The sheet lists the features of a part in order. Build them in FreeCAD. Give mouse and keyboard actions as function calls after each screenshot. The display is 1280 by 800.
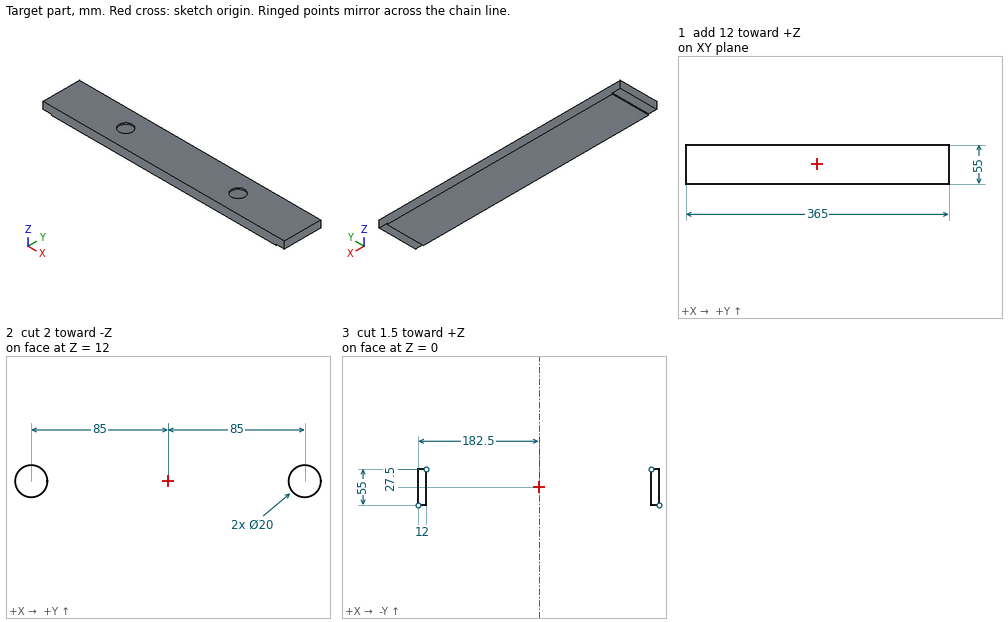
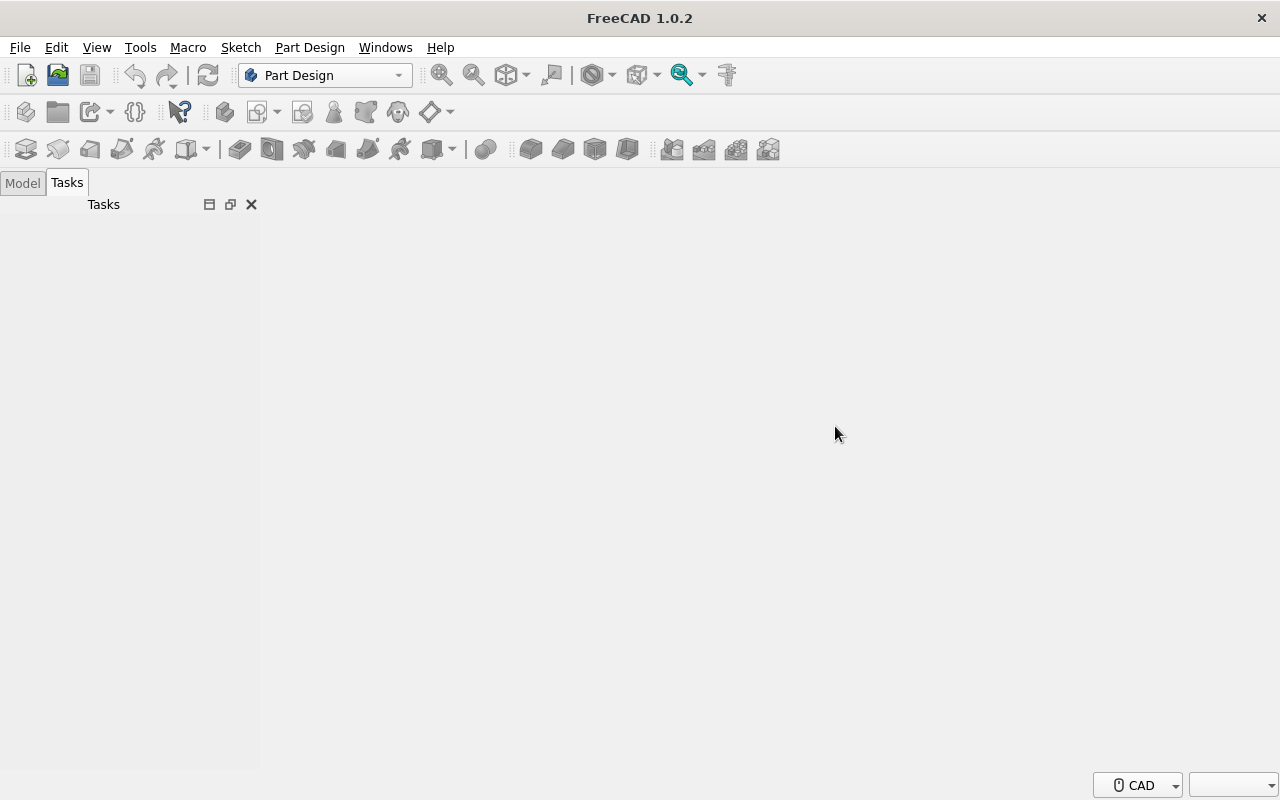
key(ctrl+n)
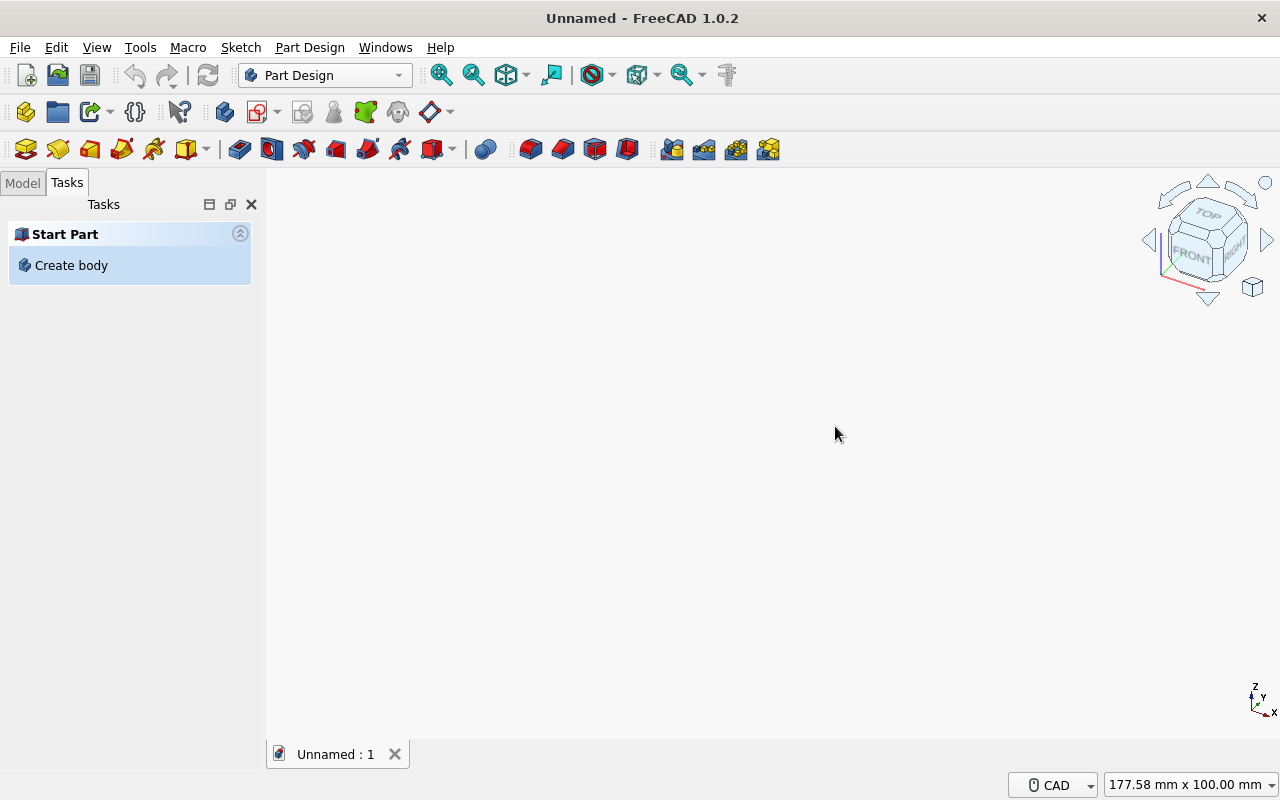
click(258, 112)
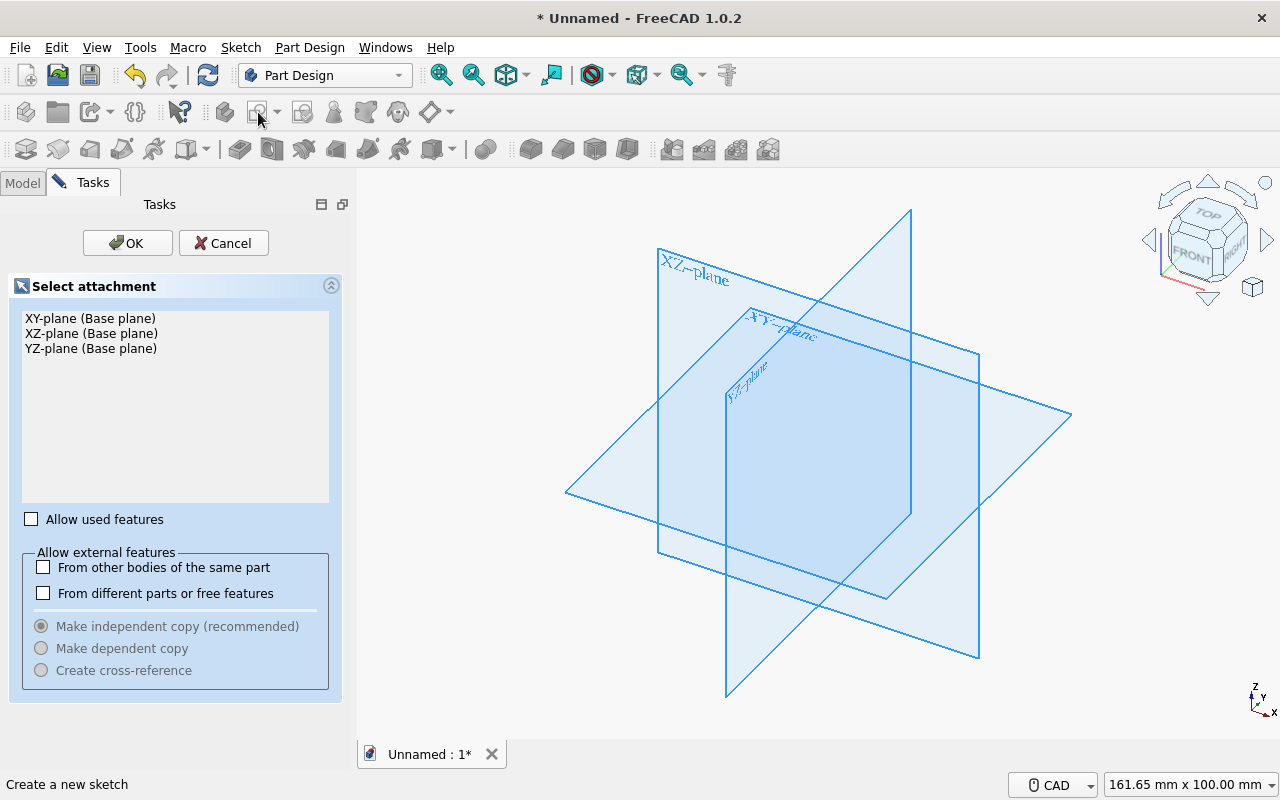
click(82, 318)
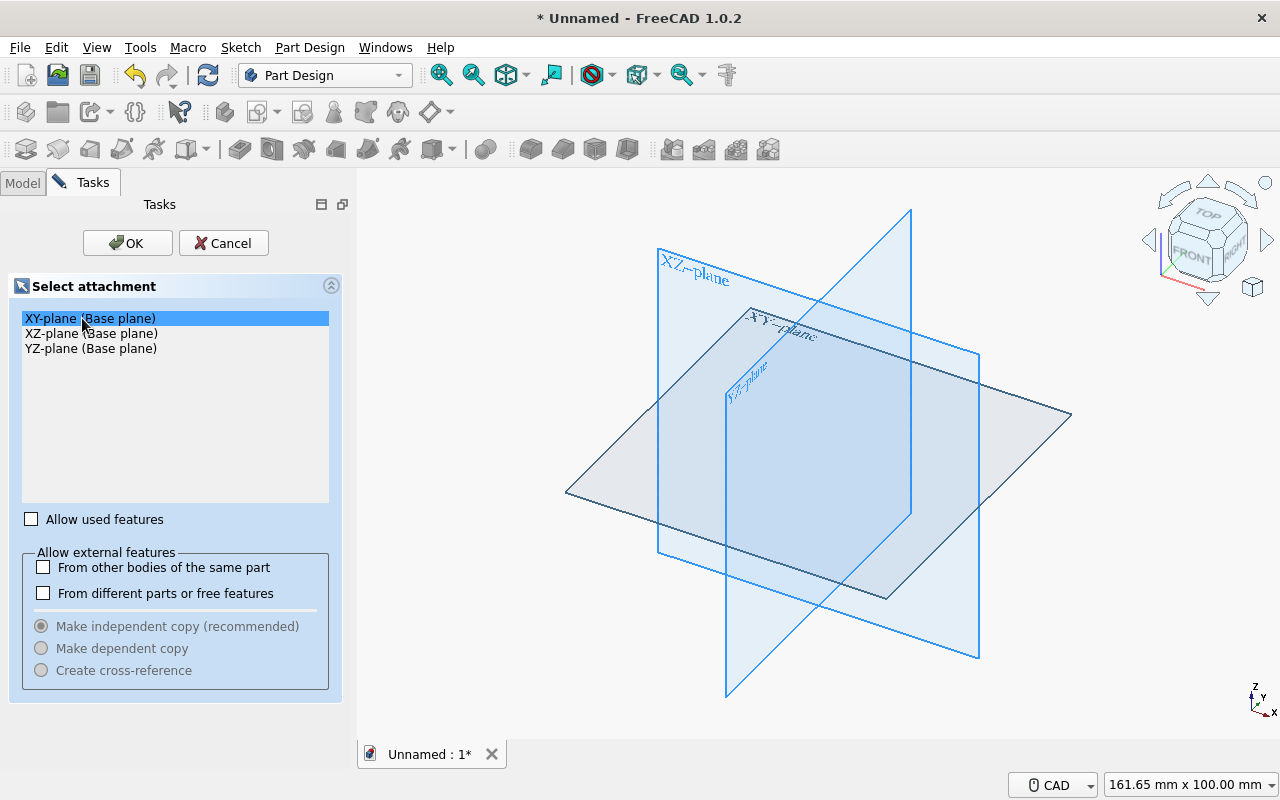
click(128, 243)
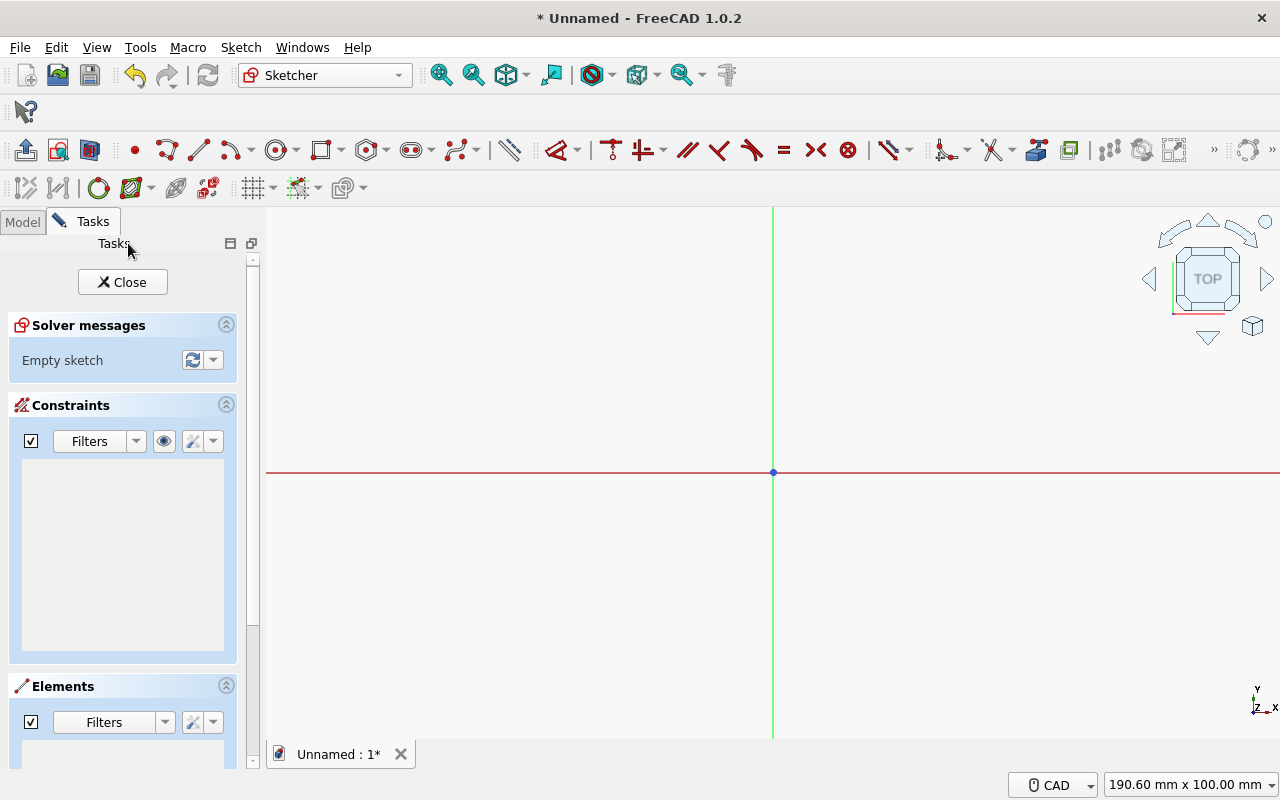
scroll(675, 473, down, 6)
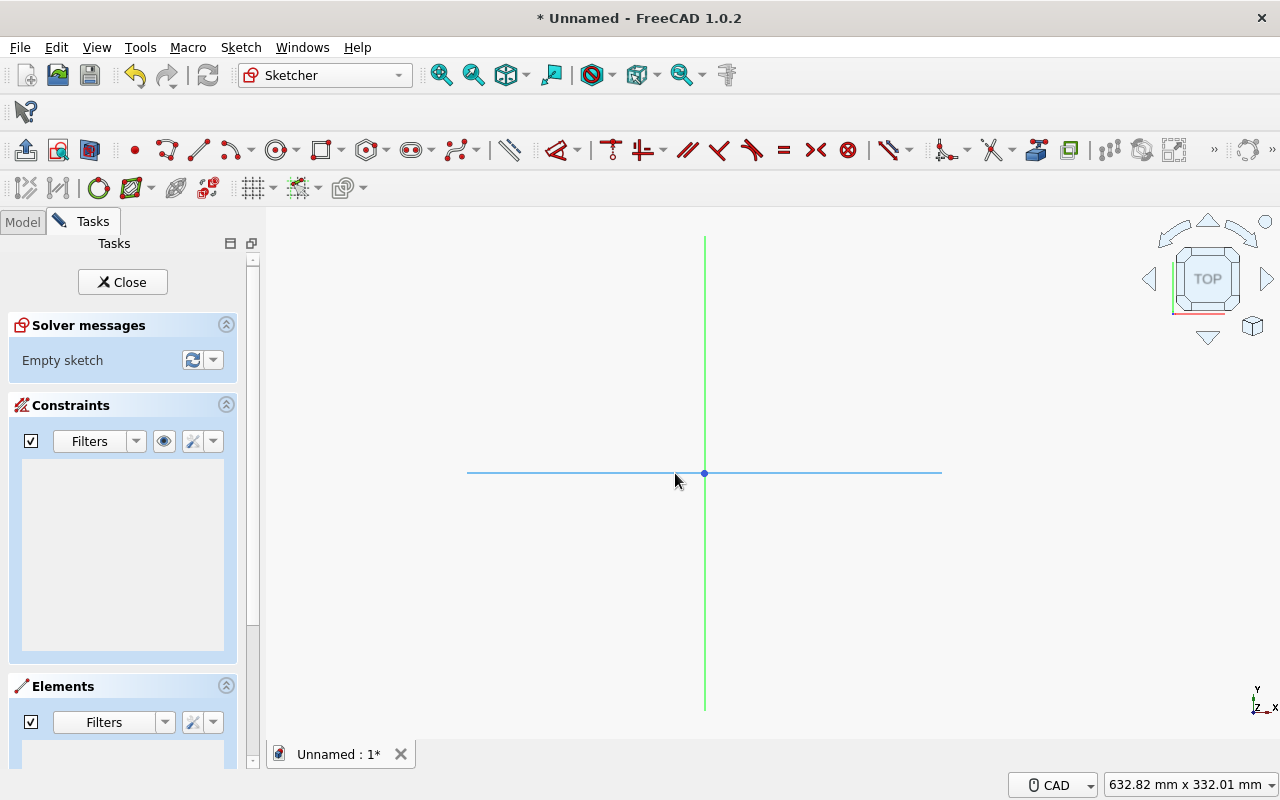
key(g)
key(v)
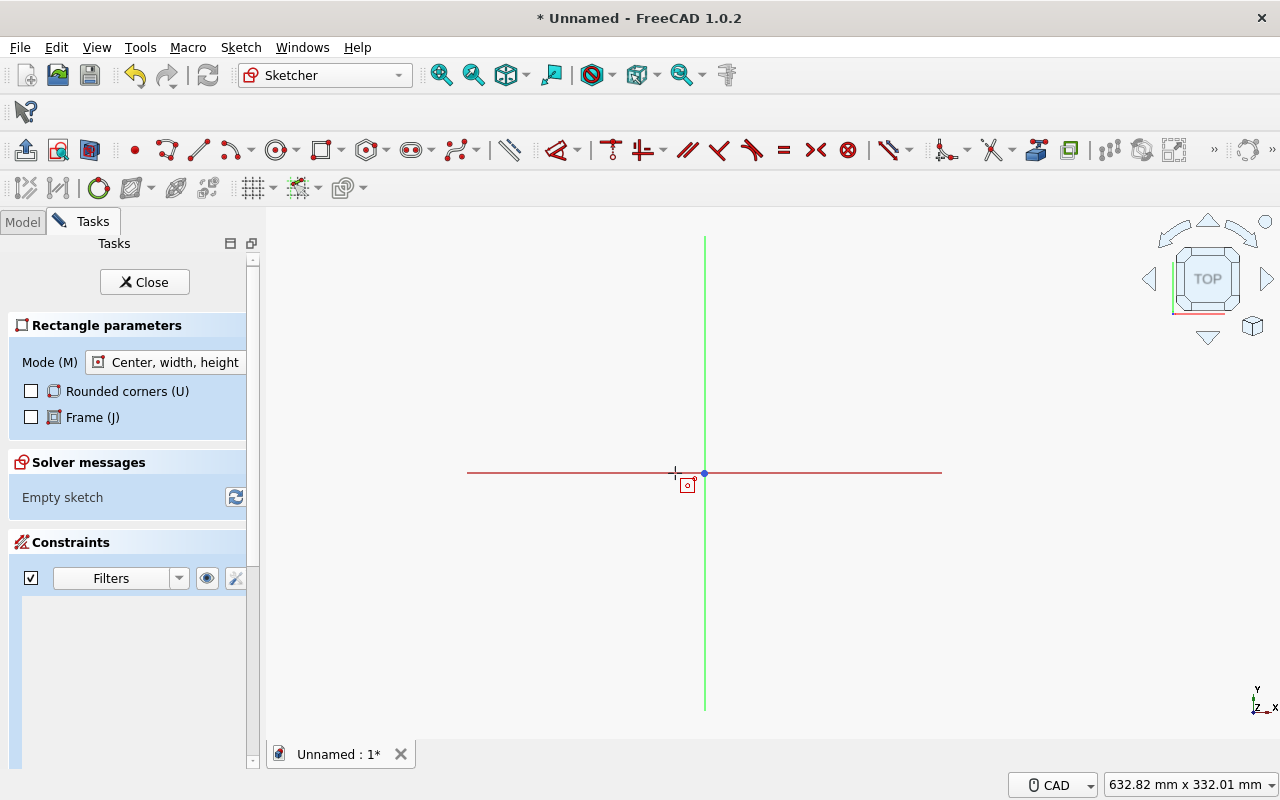
click(705, 473)
click(997, 429)
key(Escape)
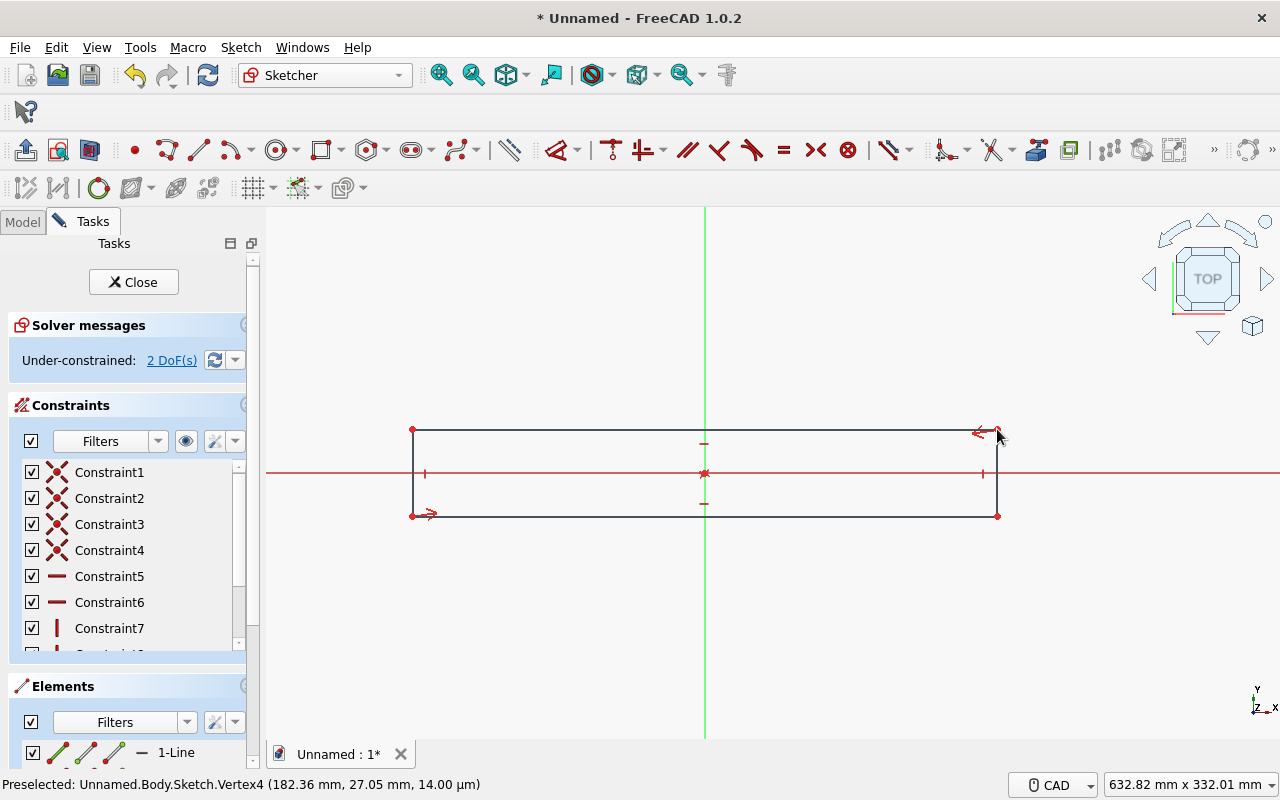
key(d)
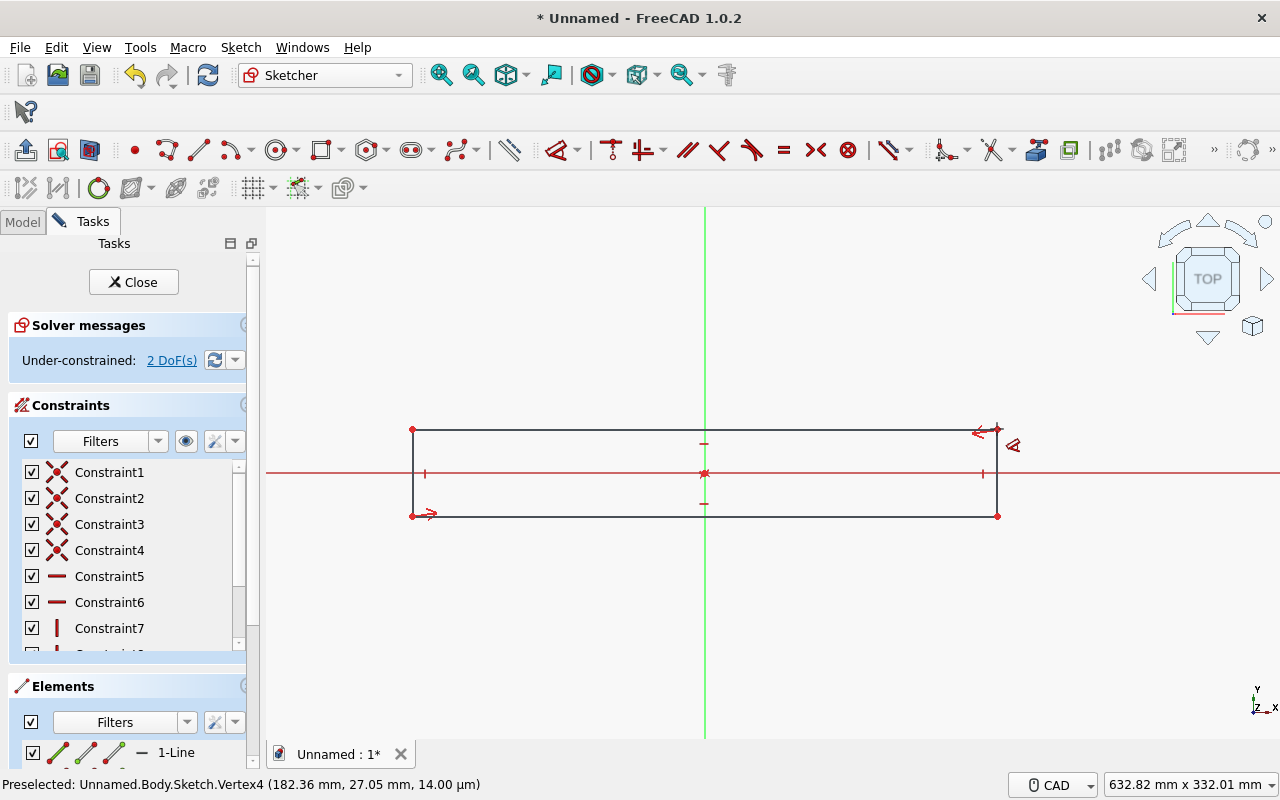
click(997, 491)
click(1031, 453)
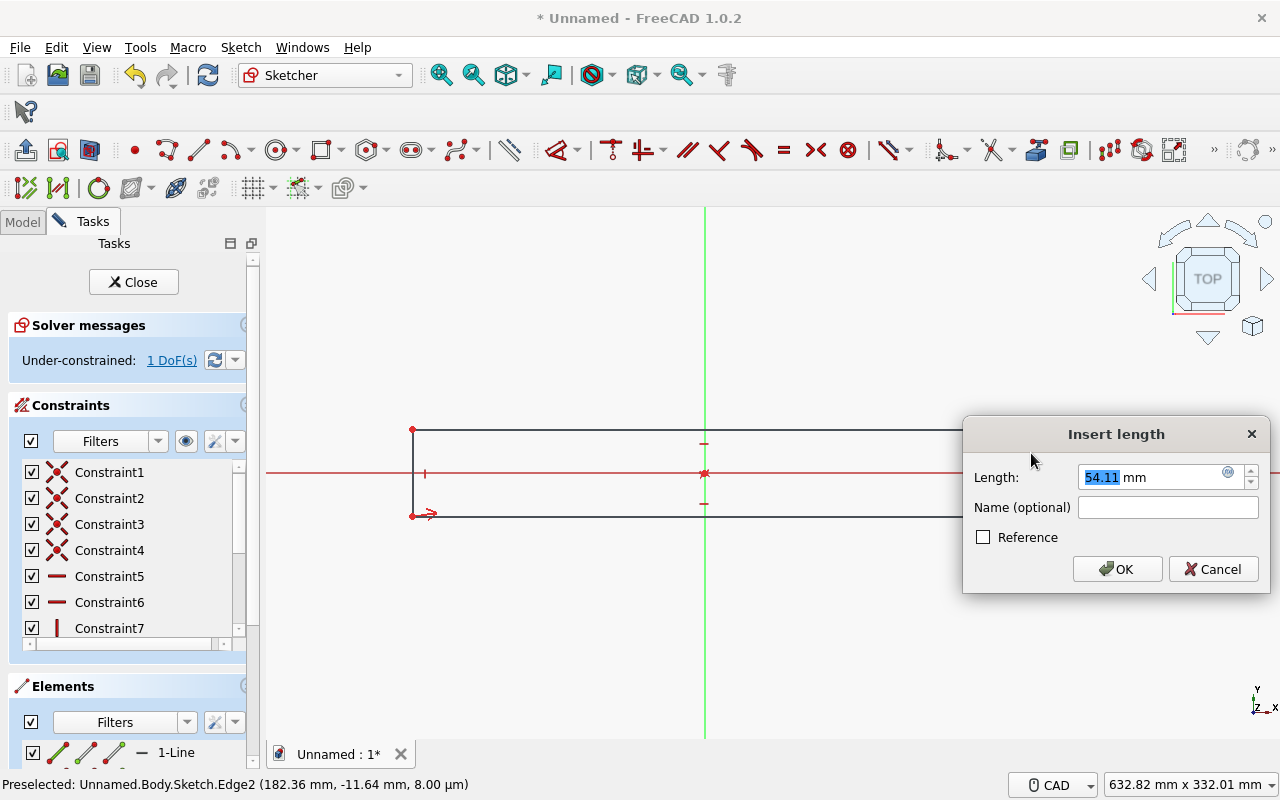
text(55)
key(Return)